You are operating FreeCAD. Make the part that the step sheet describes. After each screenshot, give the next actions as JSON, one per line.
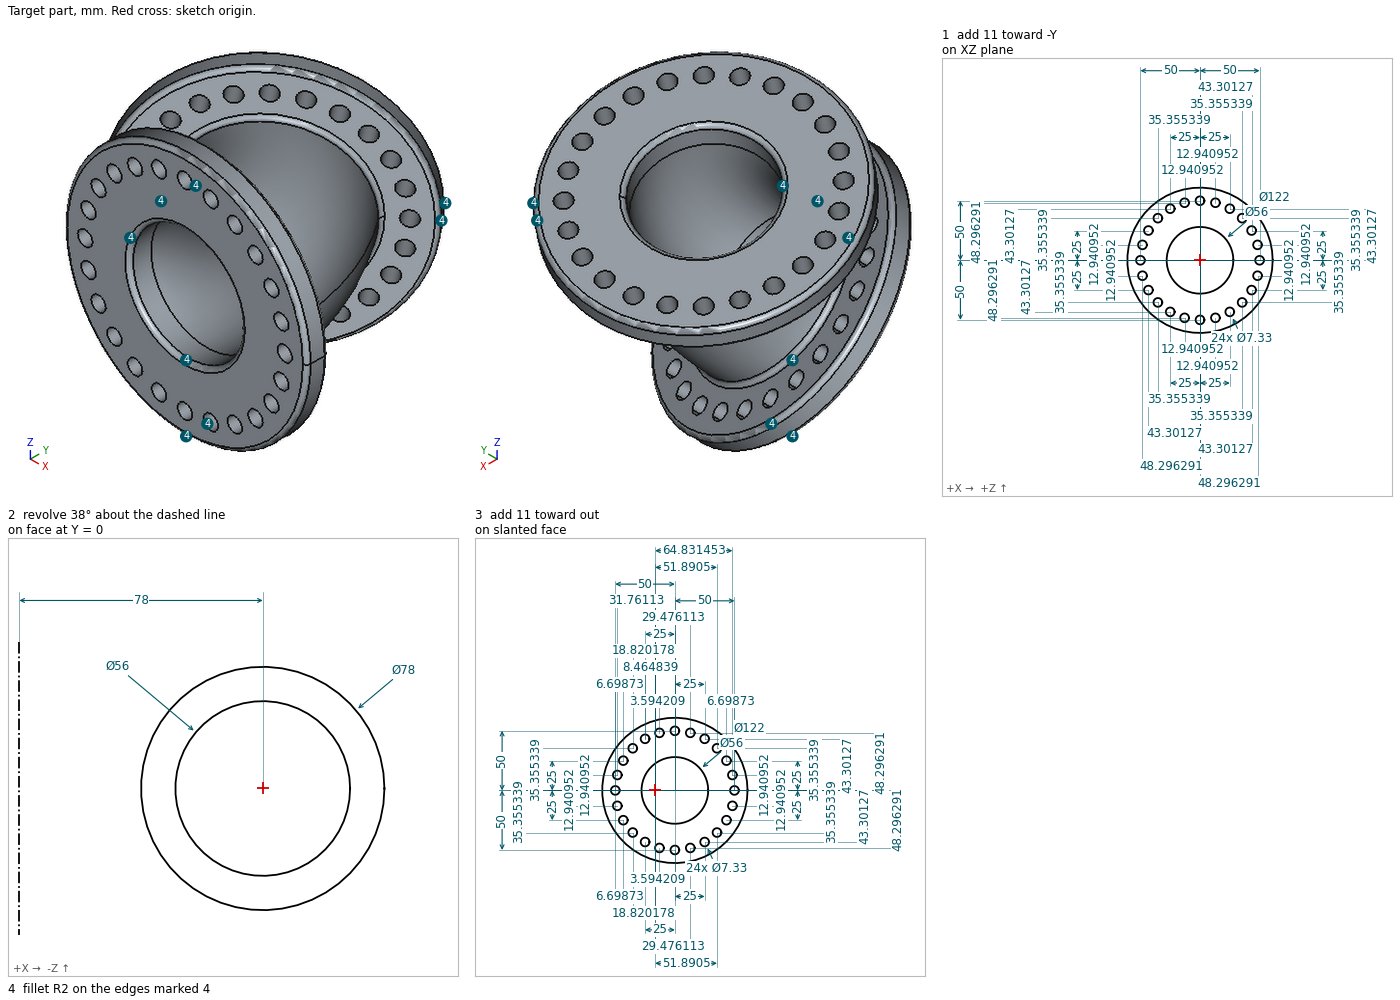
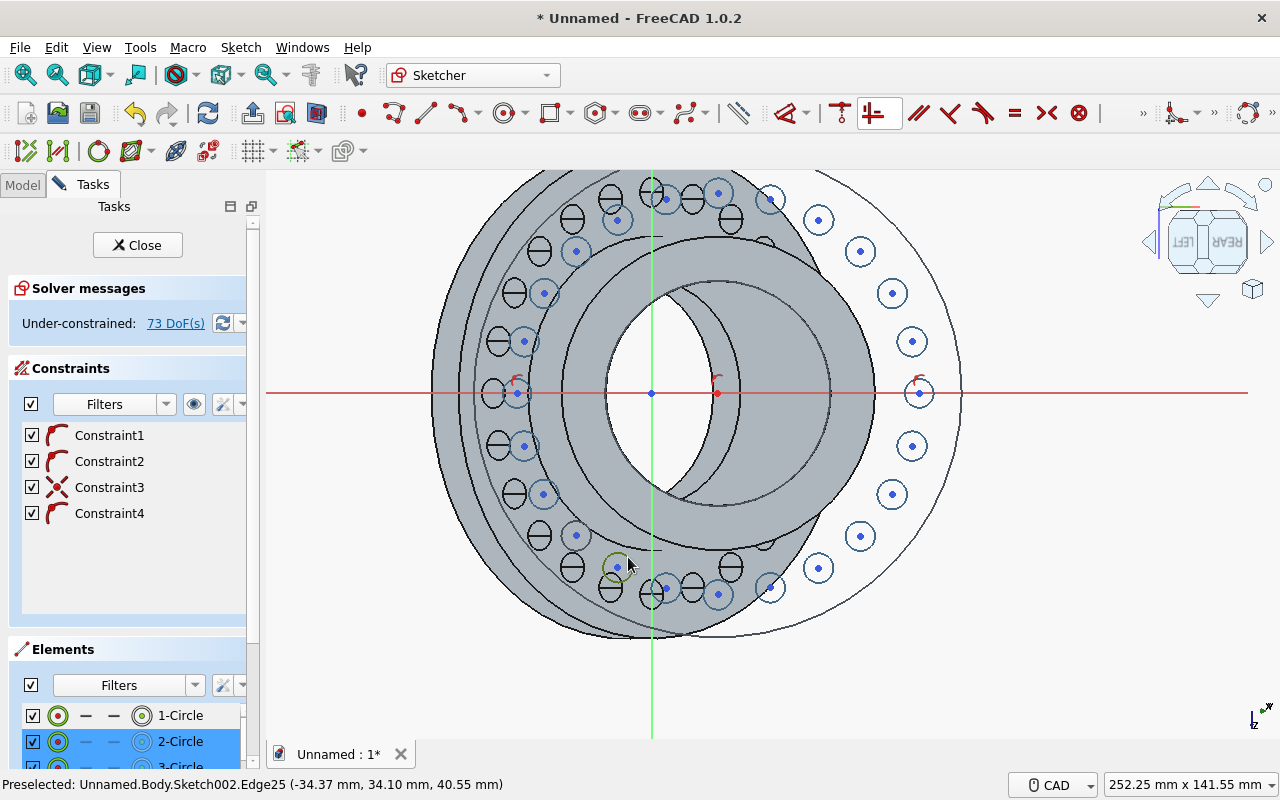
{"action": "left_click", "coordinate": [587, 525]}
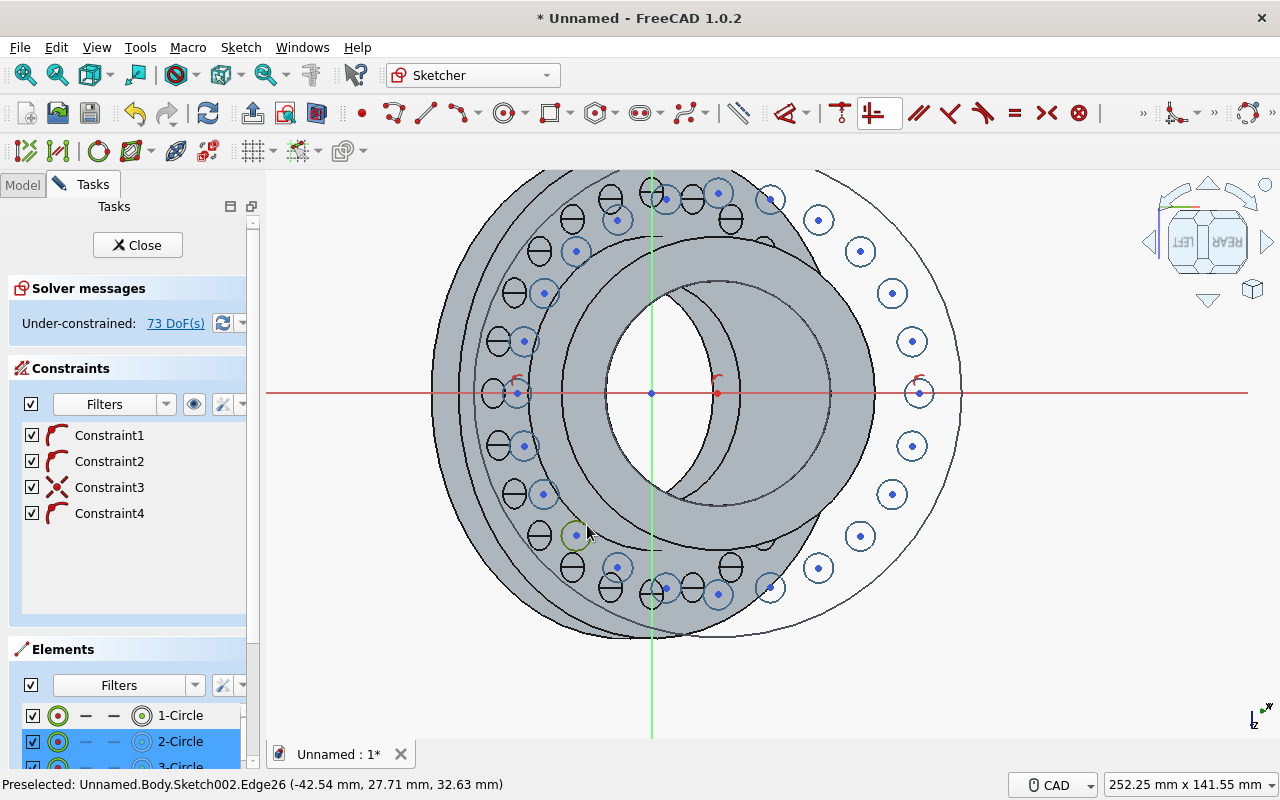
{"action": "left_click", "coordinate": [1016, 114]}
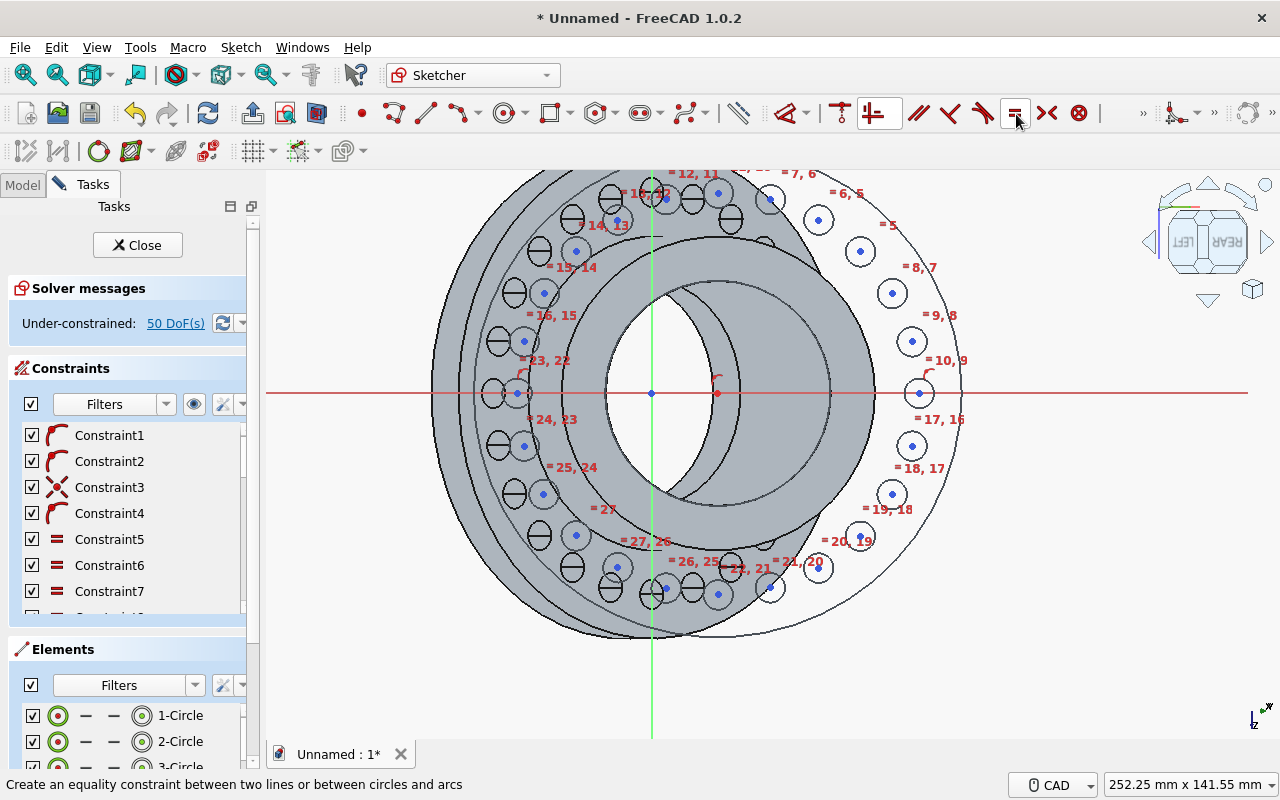
{"action": "left_click", "coordinate": [718, 393]}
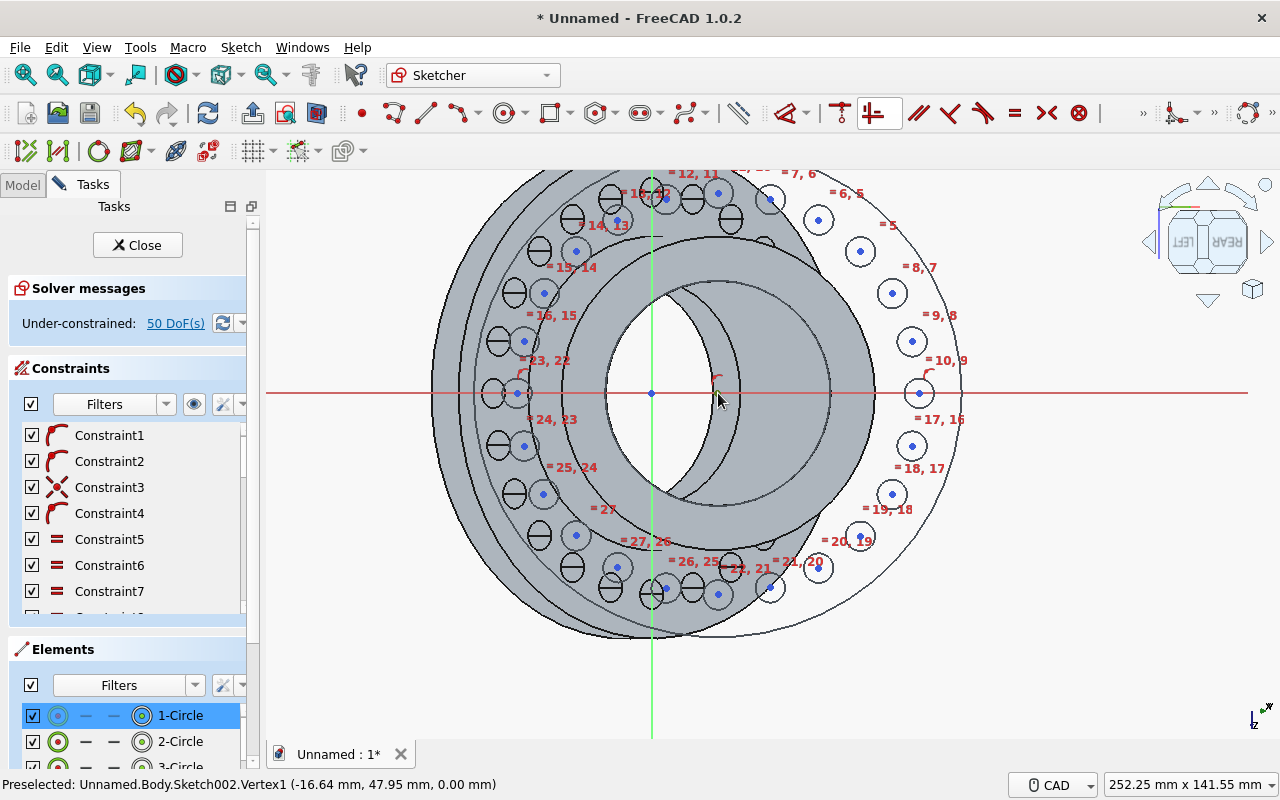
{"action": "scroll", "coordinate": [677, 579], "scroll_direction": "down", "scroll_amount": 2}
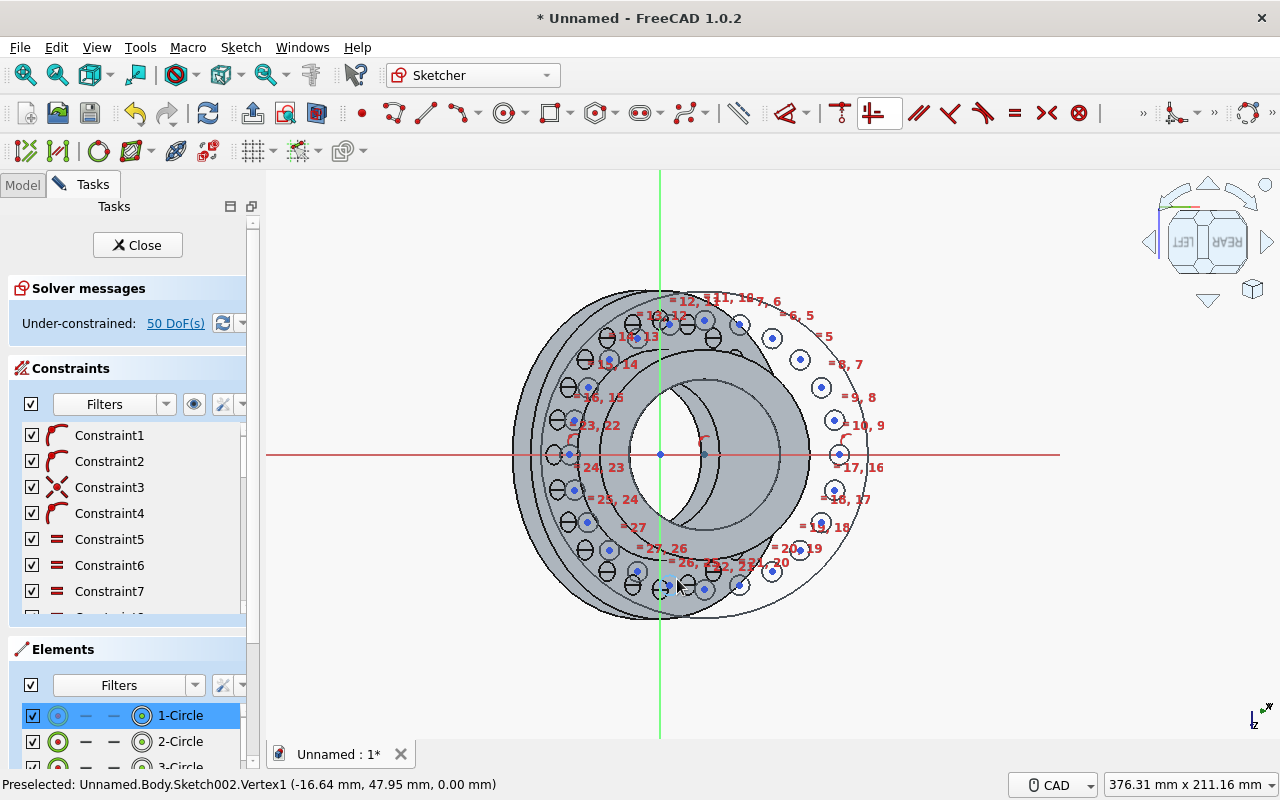
{"action": "left_click", "coordinate": [705, 321]}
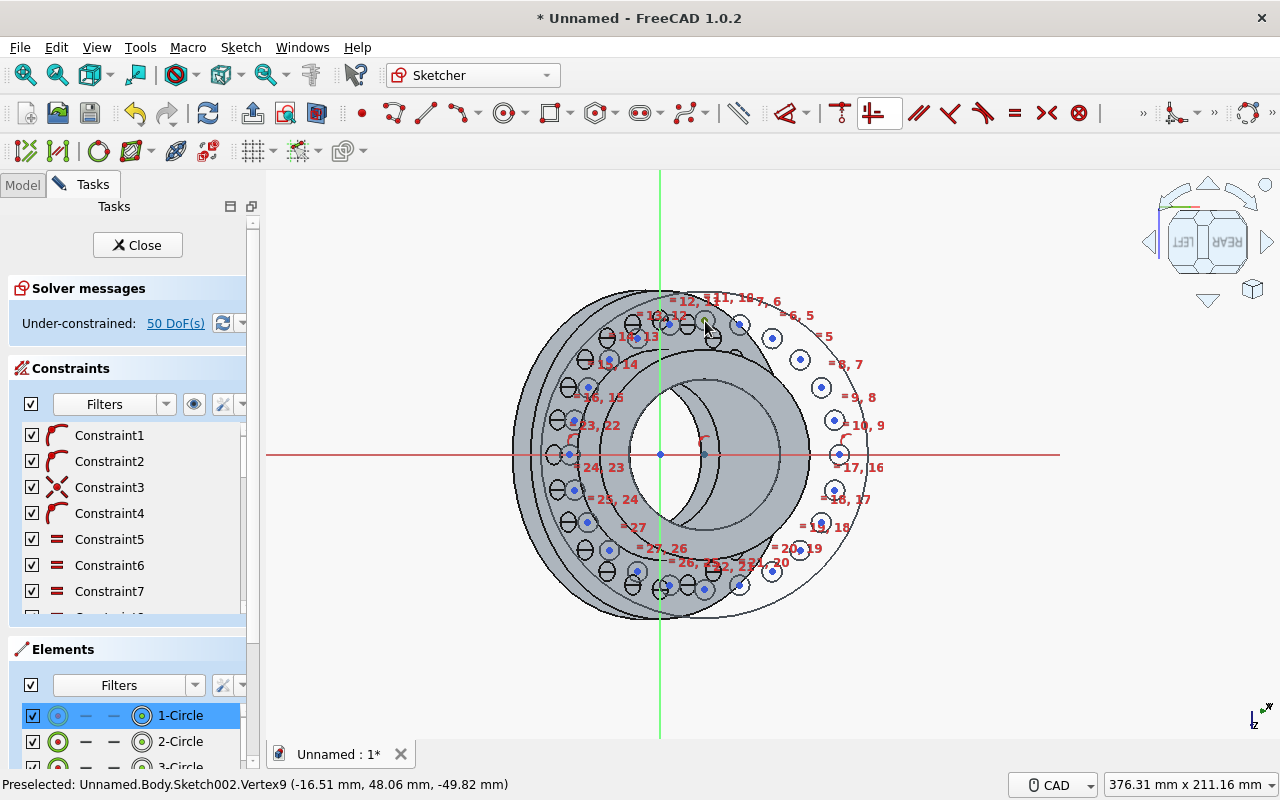
{"action": "left_click", "coordinate": [896, 114]}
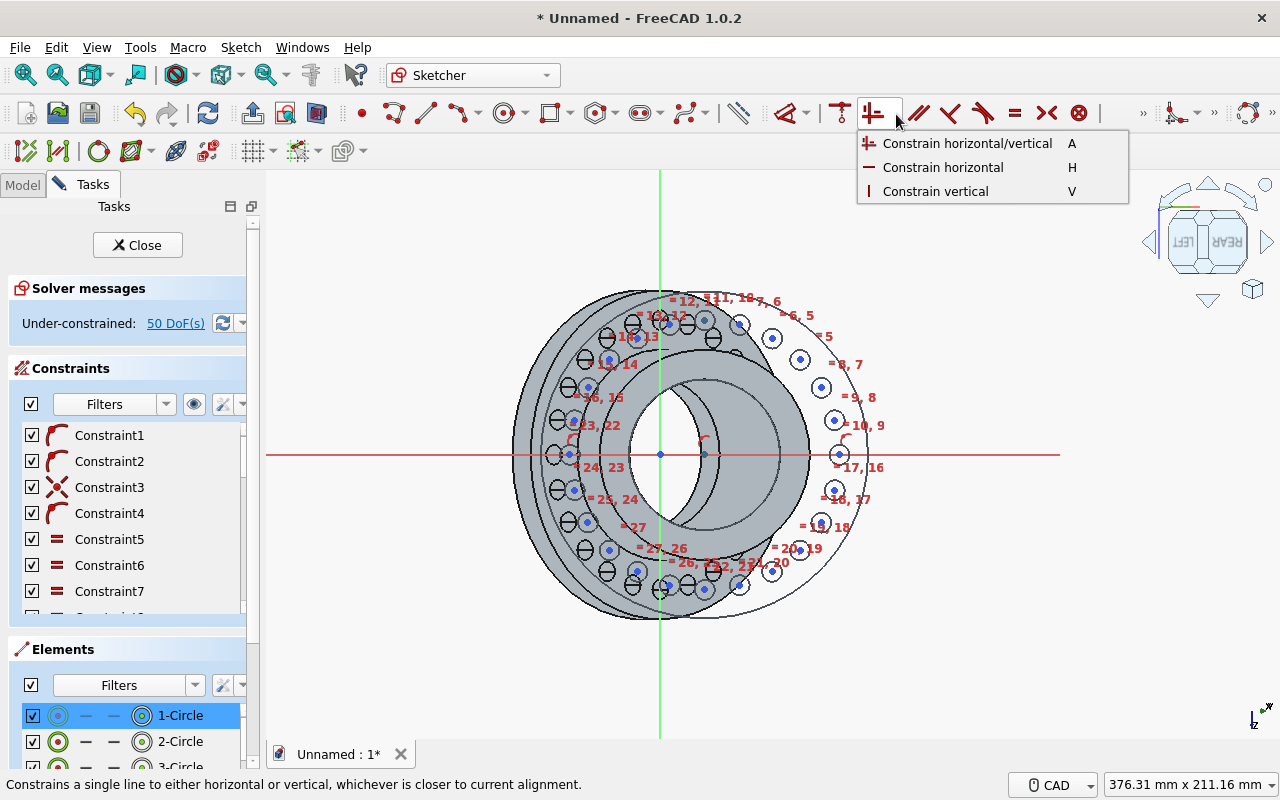
{"action": "left_click", "coordinate": [993, 191]}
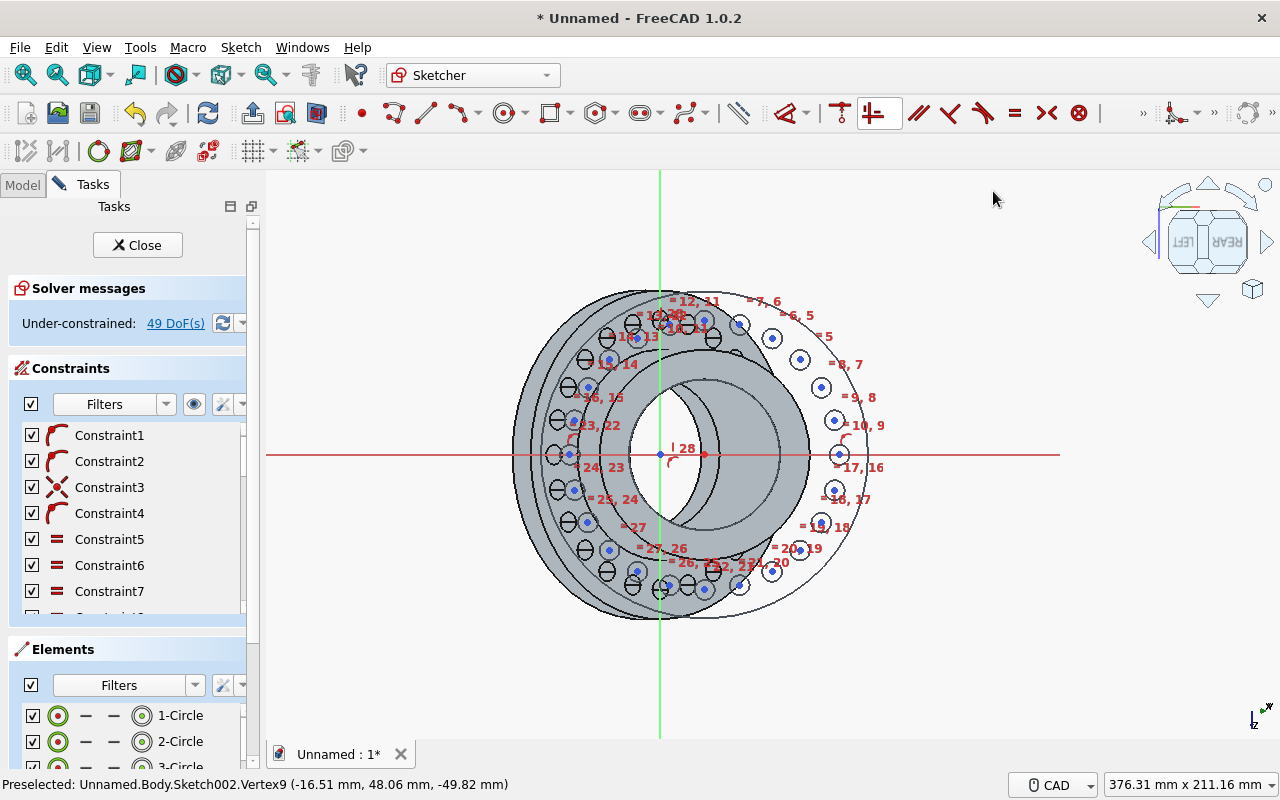
{"action": "left_click", "coordinate": [740, 325]}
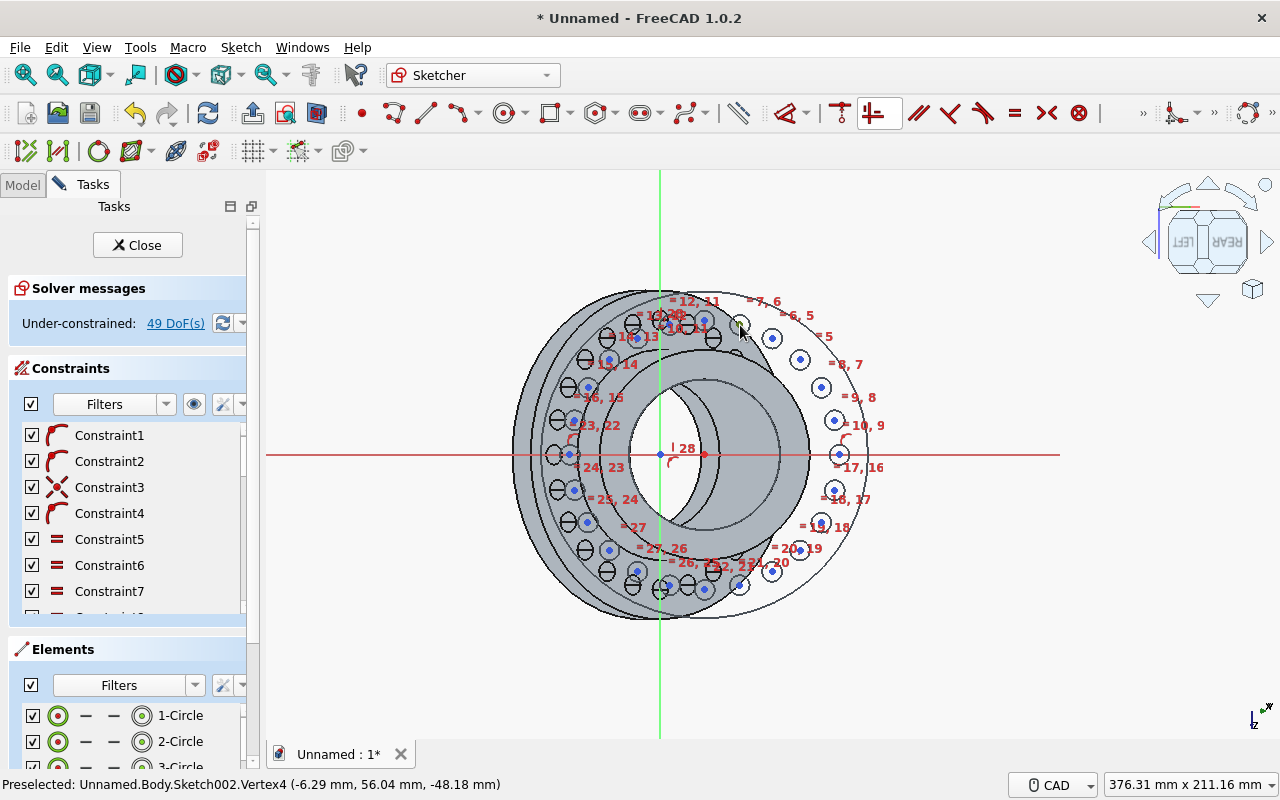
{"action": "scroll", "coordinate": [670, 325], "scroll_direction": "up", "scroll_amount": 4}